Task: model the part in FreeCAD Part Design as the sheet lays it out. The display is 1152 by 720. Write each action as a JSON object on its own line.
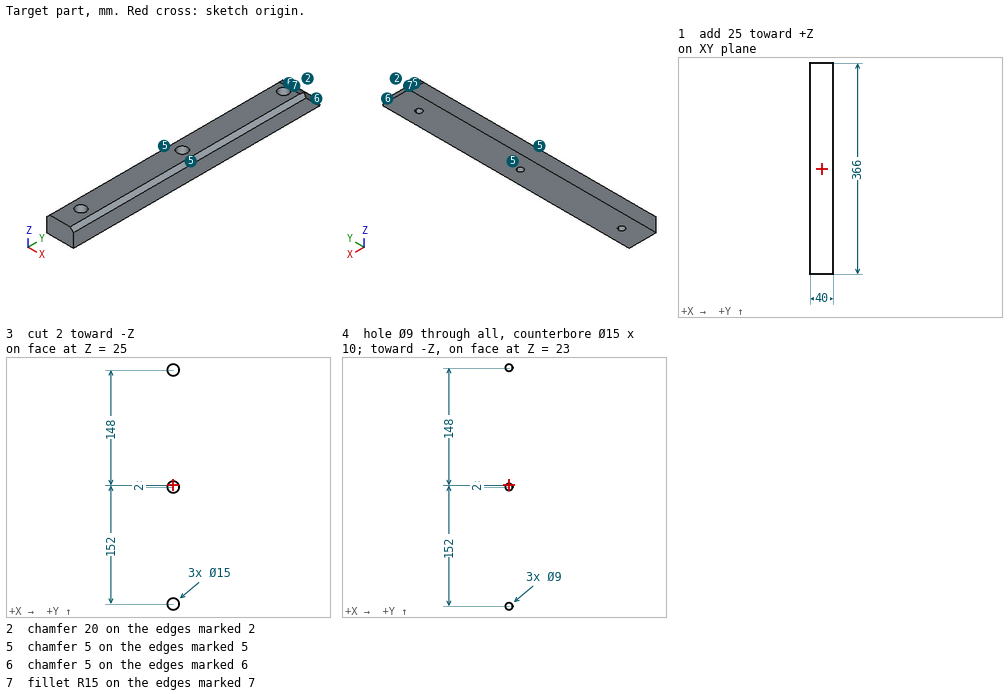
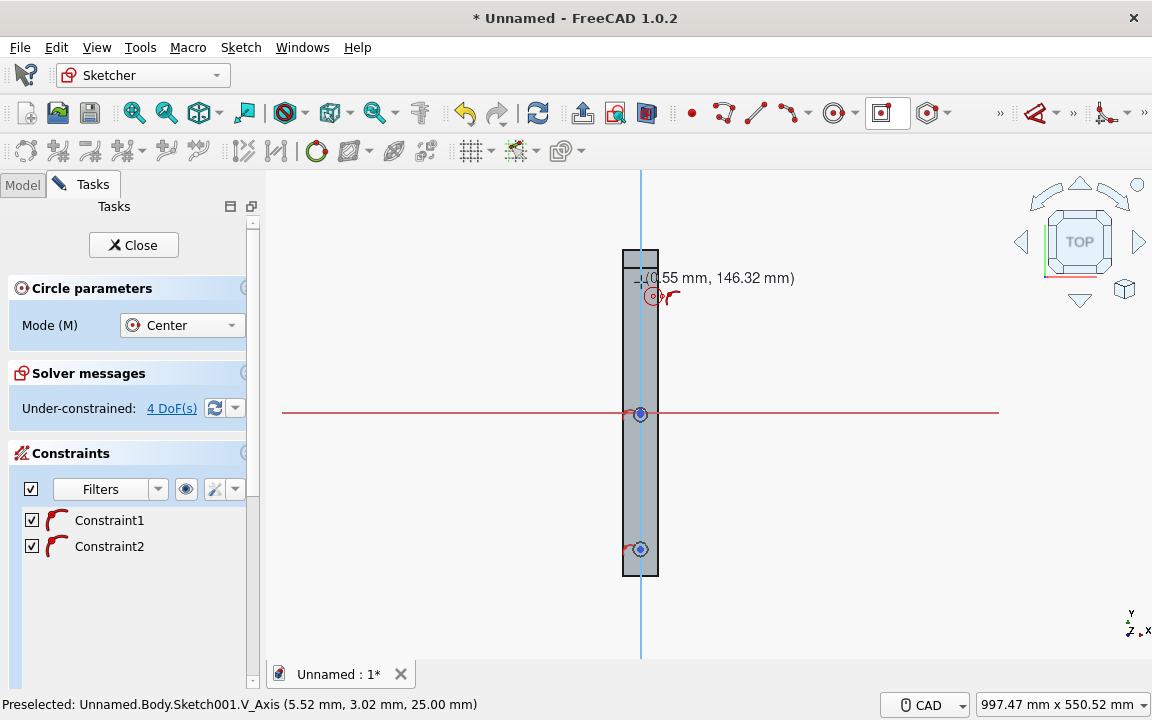
{"action": "left_click", "coordinate": [641, 282]}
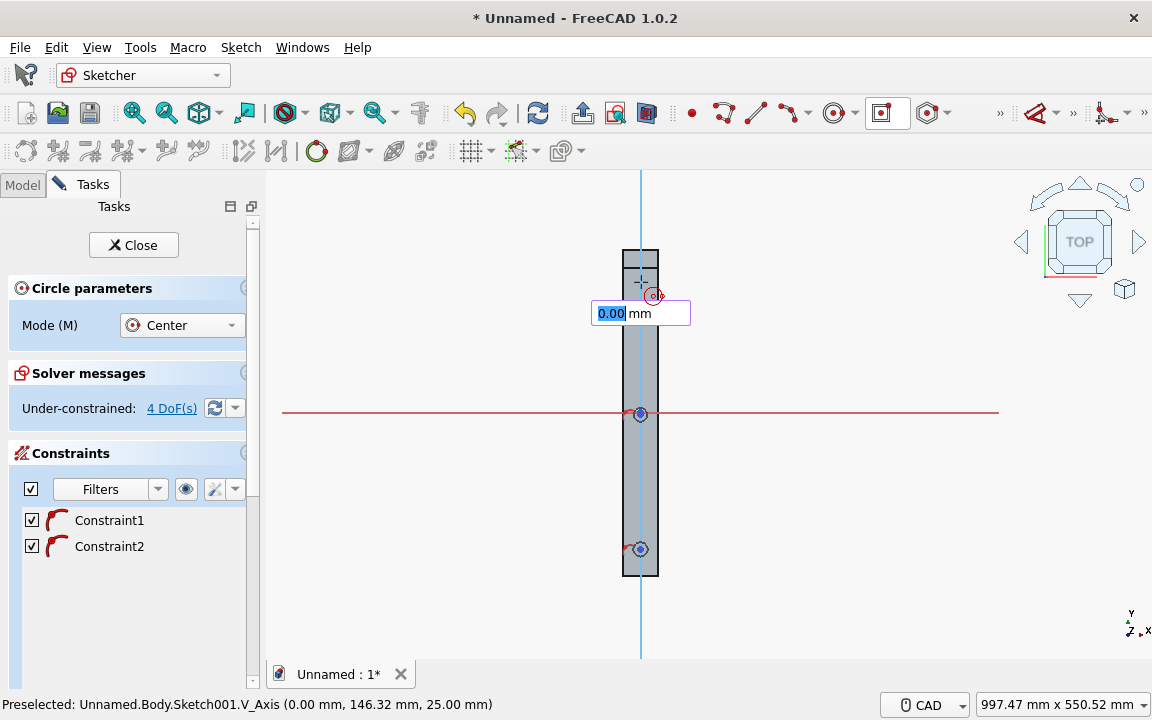
{"action": "scroll", "coordinate": [647, 279], "scroll_direction": "up", "scroll_amount": 5}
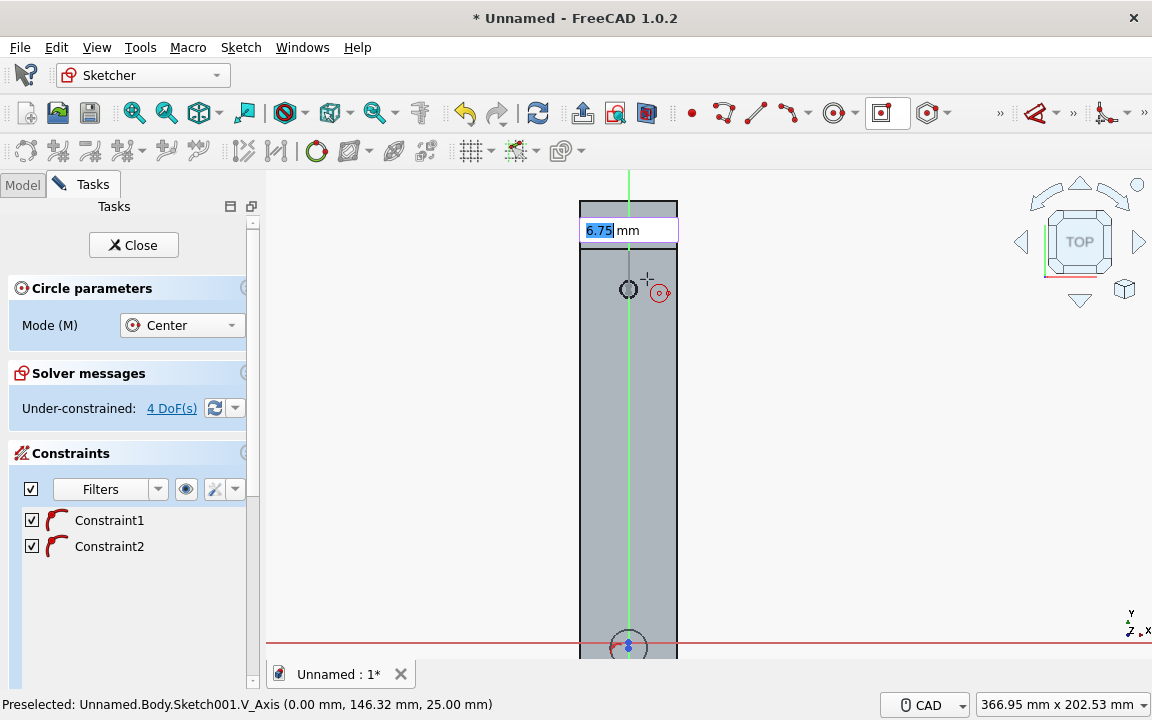
{"action": "left_click", "coordinate": [646, 279]}
{"action": "key", "text": "Escape"}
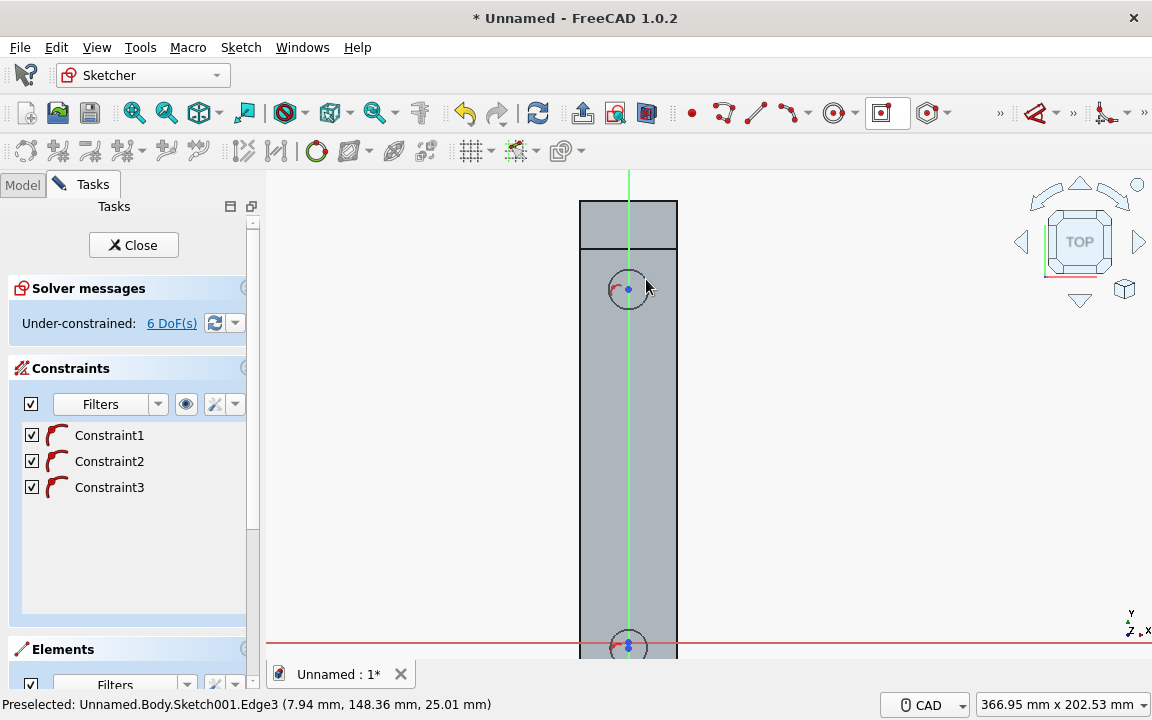
{"action": "scroll", "coordinate": [647, 279], "scroll_direction": "down", "scroll_amount": 5}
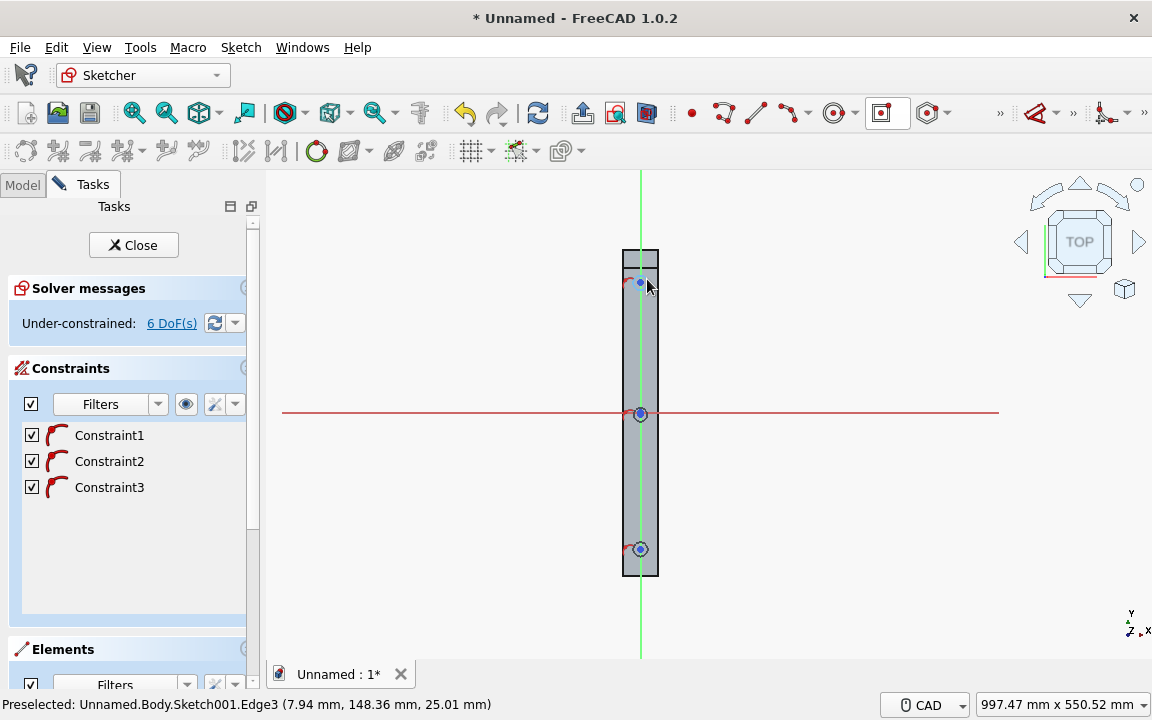
{"action": "scroll", "coordinate": [646, 544], "scroll_direction": "up", "scroll_amount": 6}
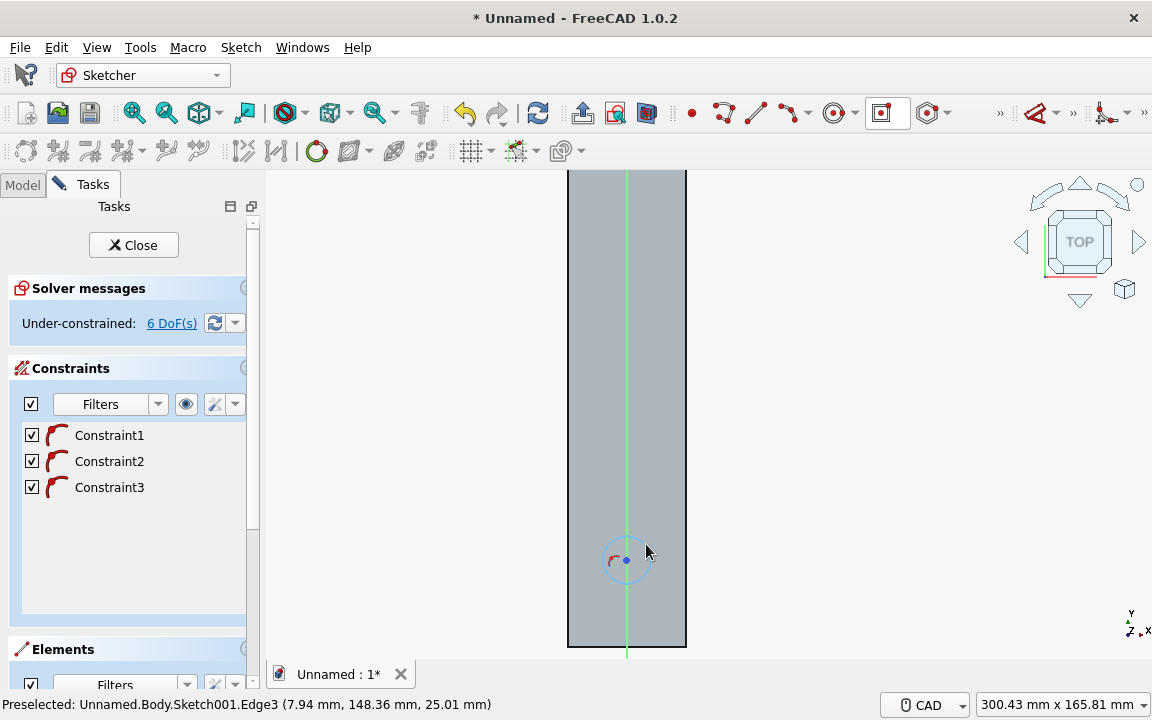
{"action": "left_click", "coordinate": [643, 543]}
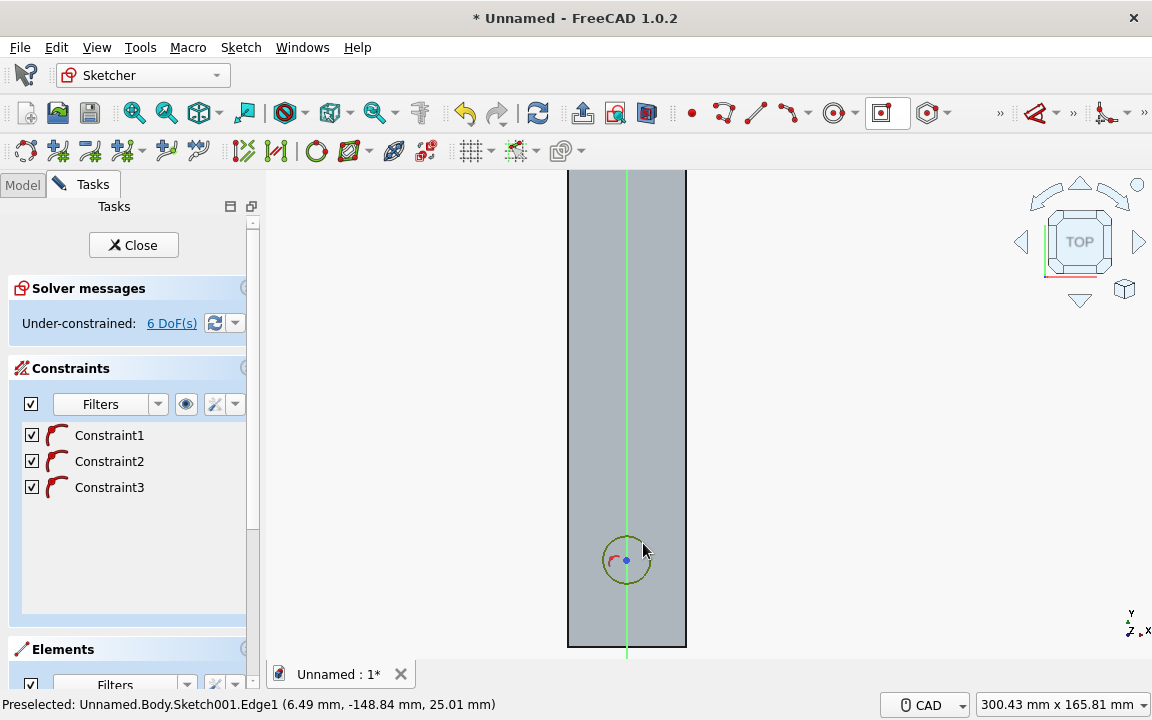
{"action": "scroll", "coordinate": [646, 544], "scroll_direction": "down", "scroll_amount": 6}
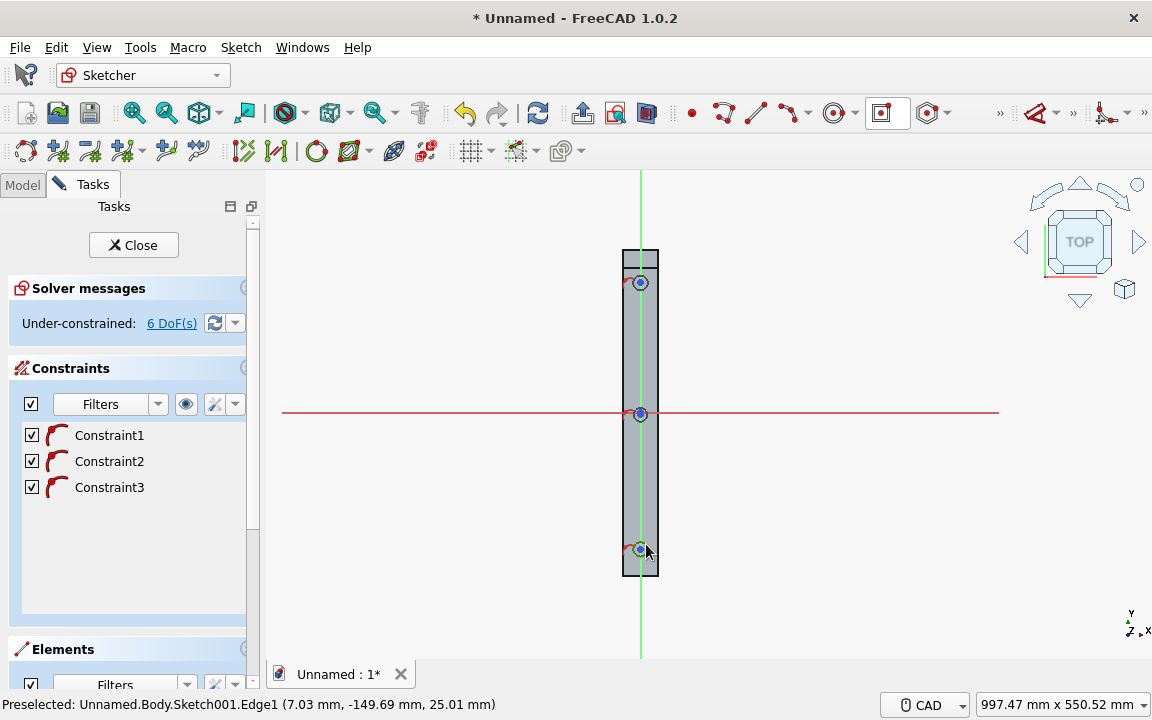
{"action": "scroll", "coordinate": [645, 410], "scroll_direction": "up", "scroll_amount": 8}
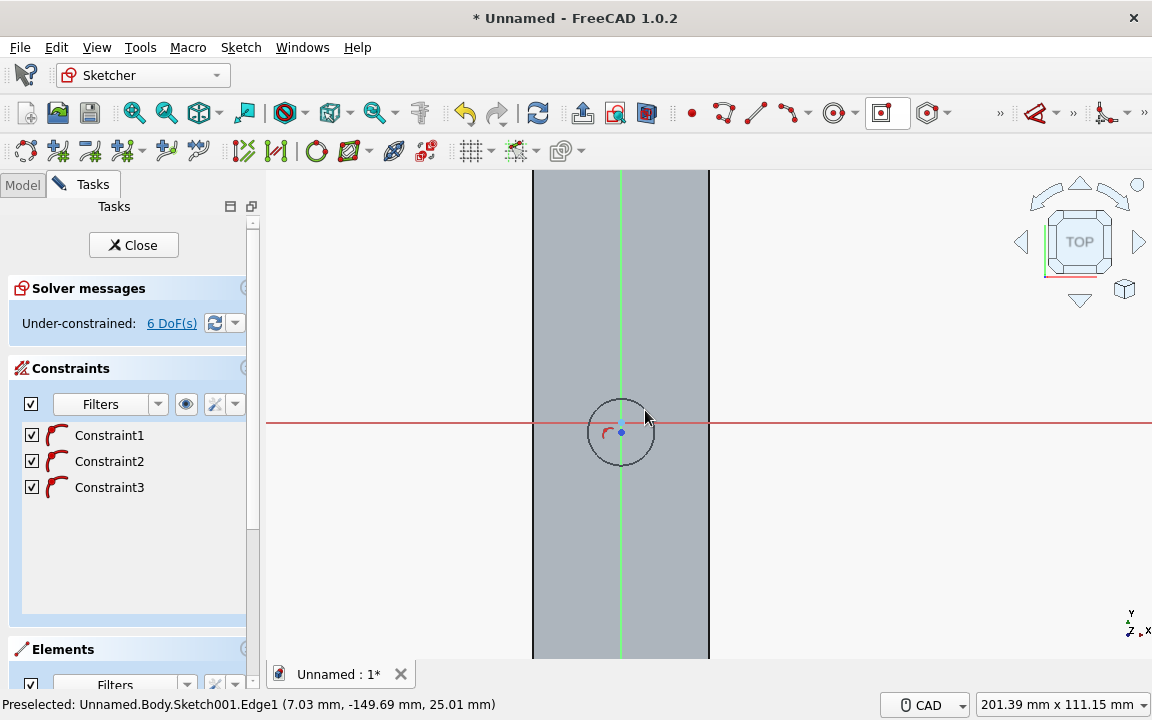
{"action": "left_click", "coordinate": [645, 409]}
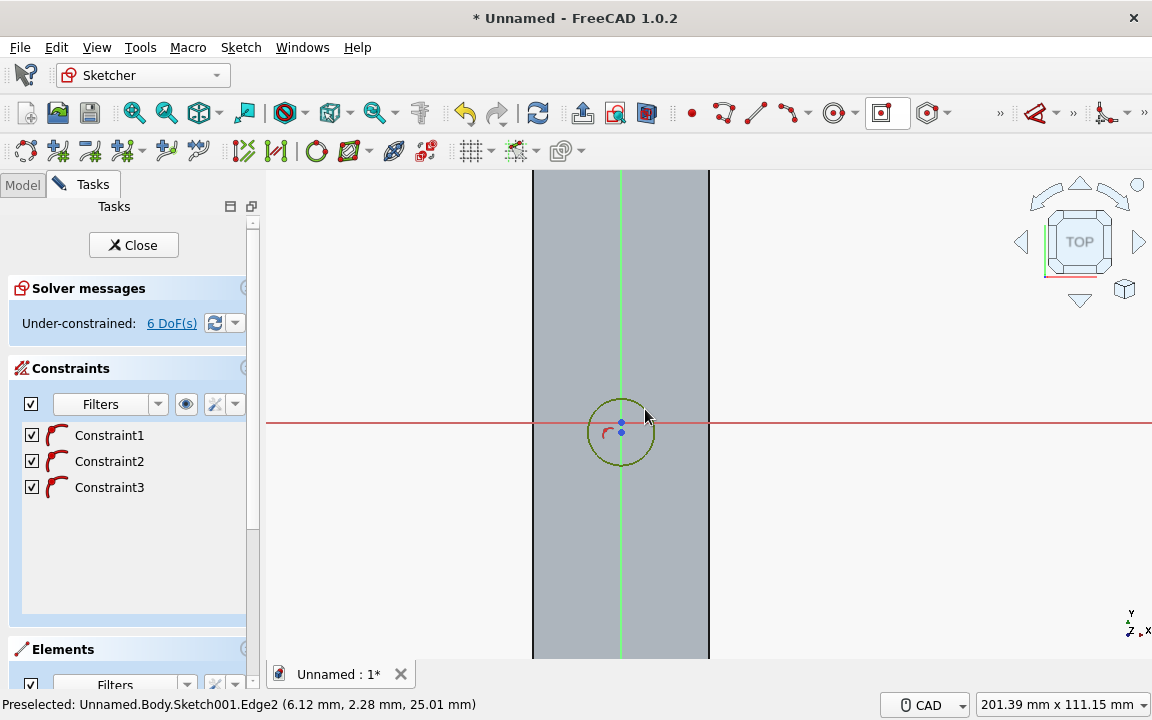
{"action": "scroll", "coordinate": [645, 410], "scroll_direction": "down", "scroll_amount": 8}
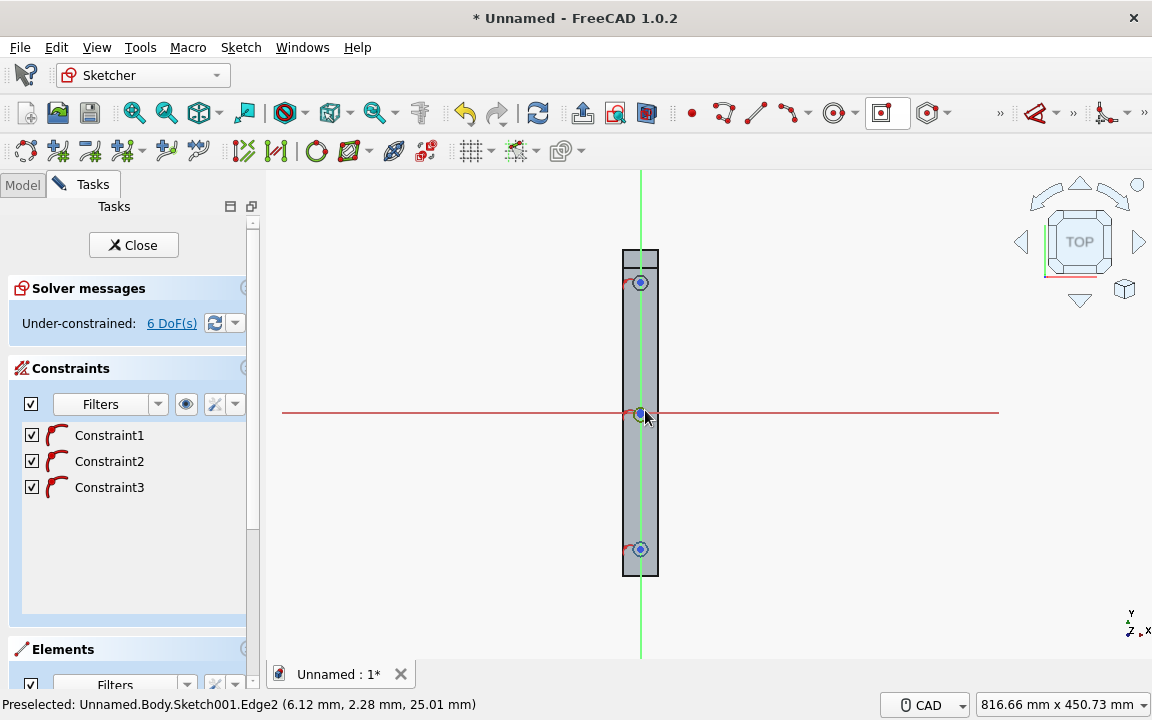
{"action": "scroll", "coordinate": [646, 278], "scroll_direction": "up", "scroll_amount": 5}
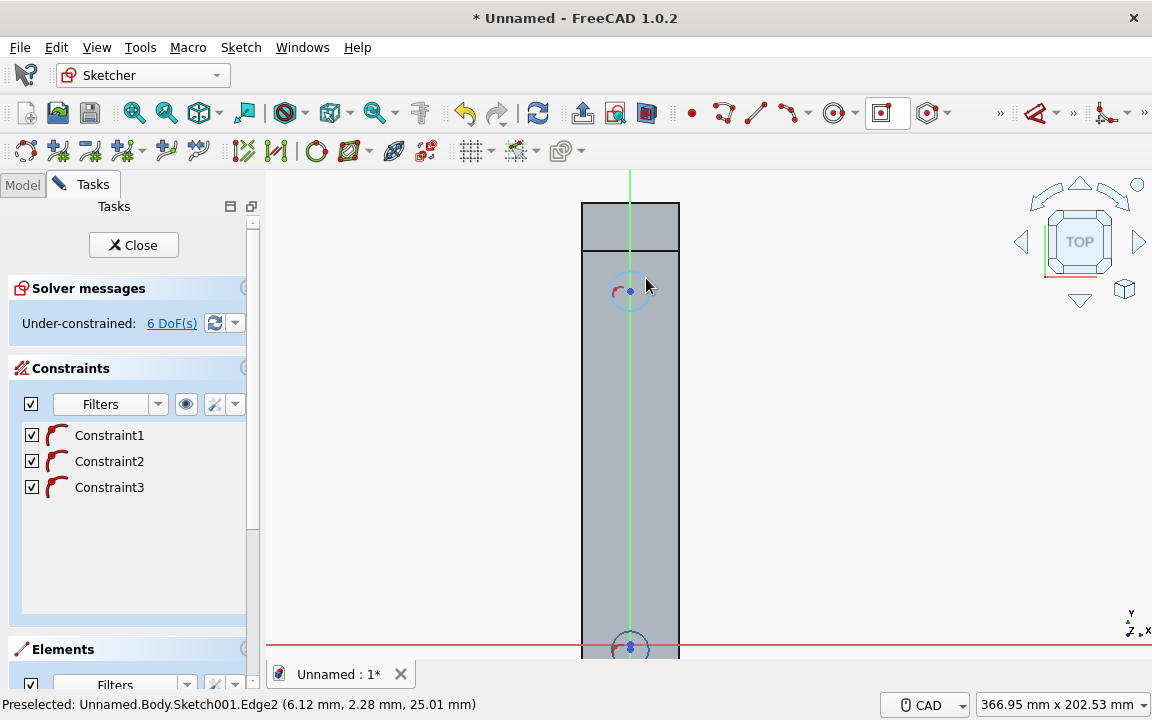
{"action": "left_click", "coordinate": [644, 277]}